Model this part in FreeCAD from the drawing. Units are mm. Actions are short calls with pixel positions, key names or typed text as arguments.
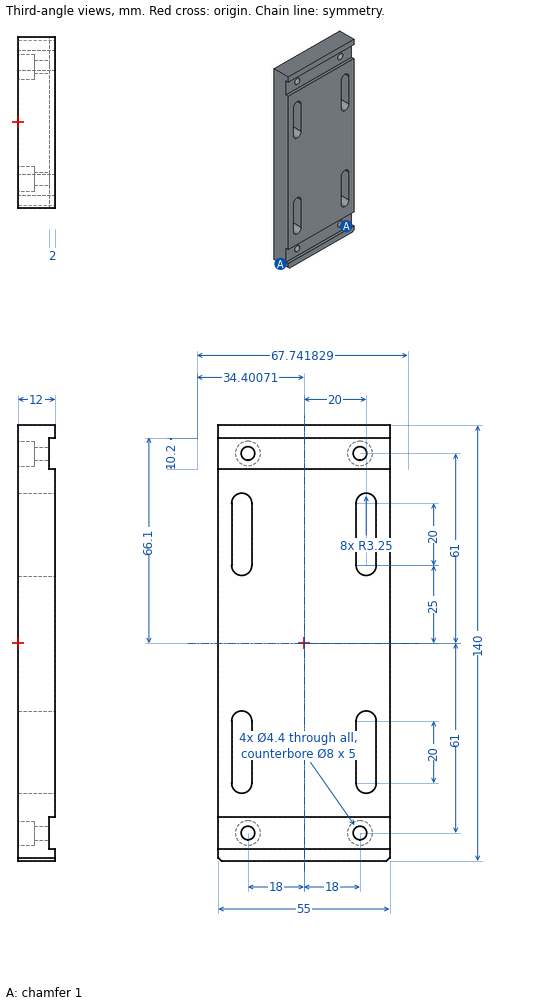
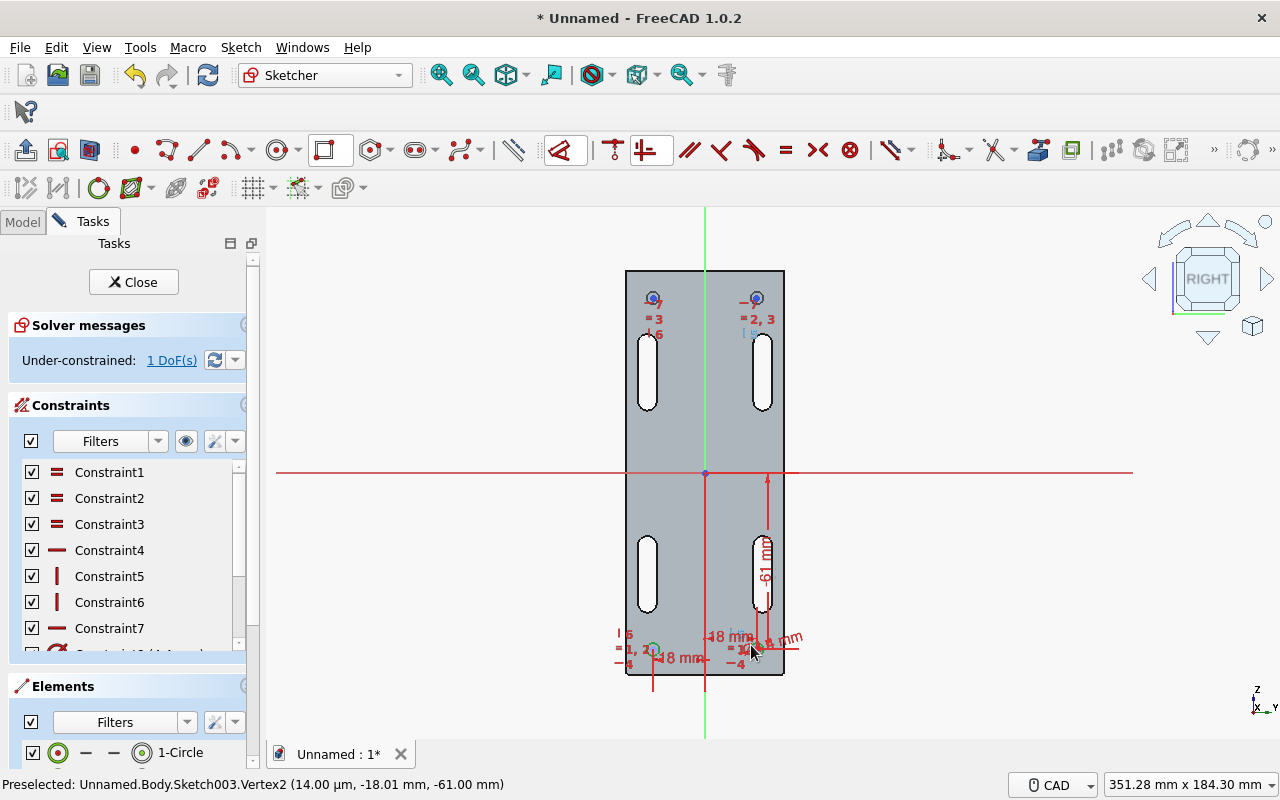
click(757, 298)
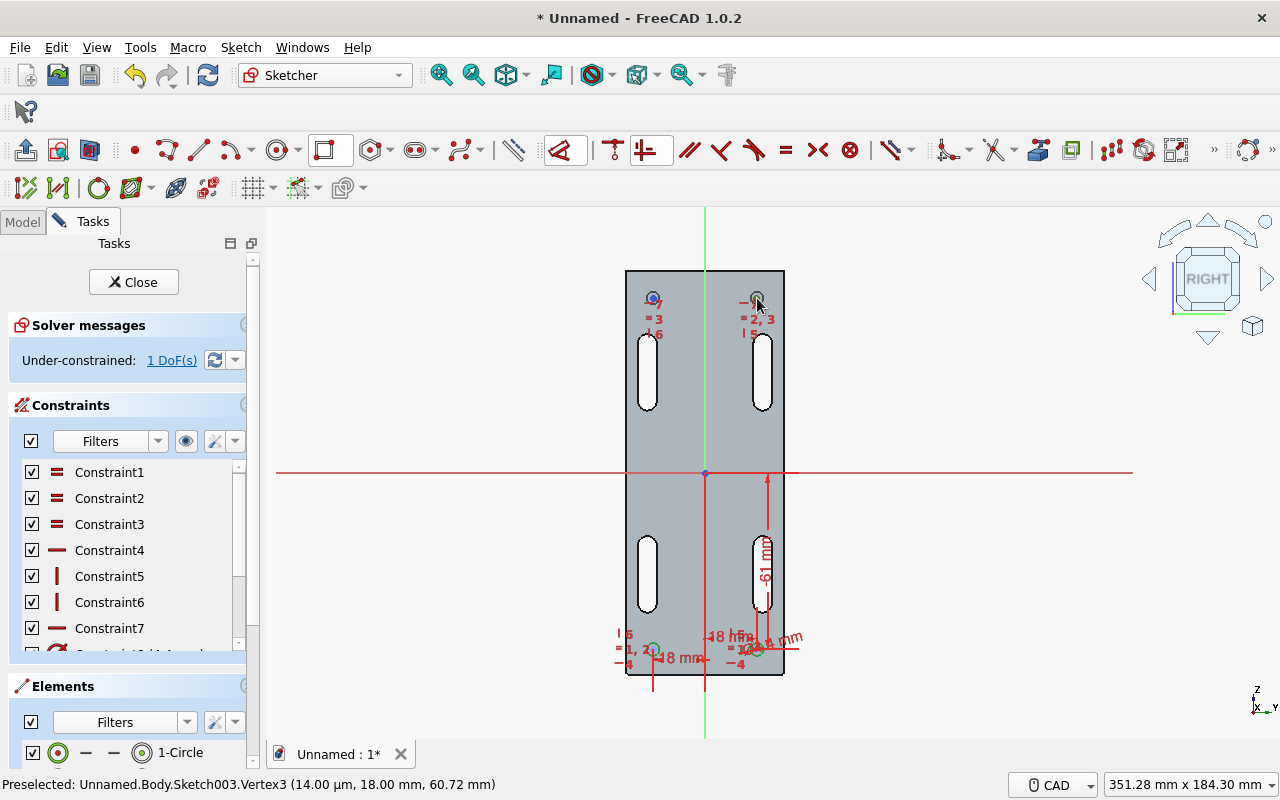
click(582, 150)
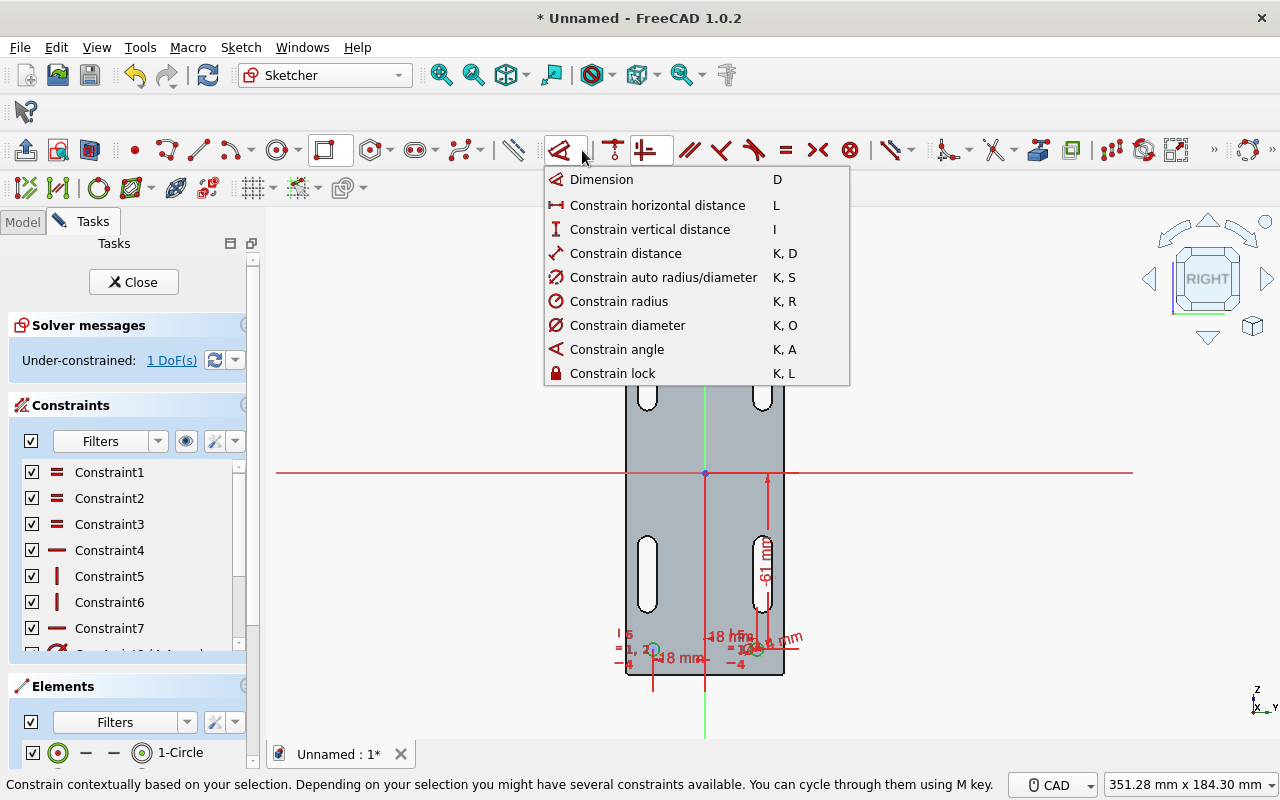
click(697, 229)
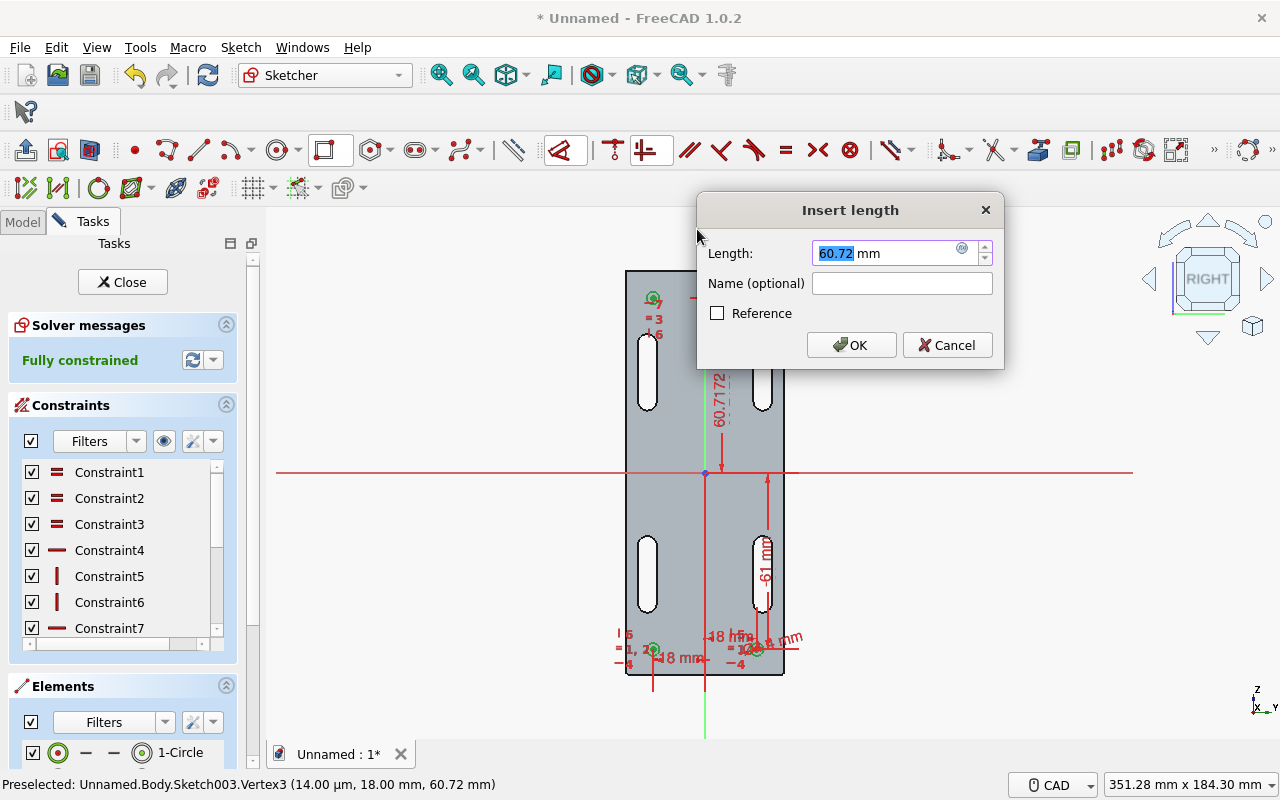
text(61)
key(Return)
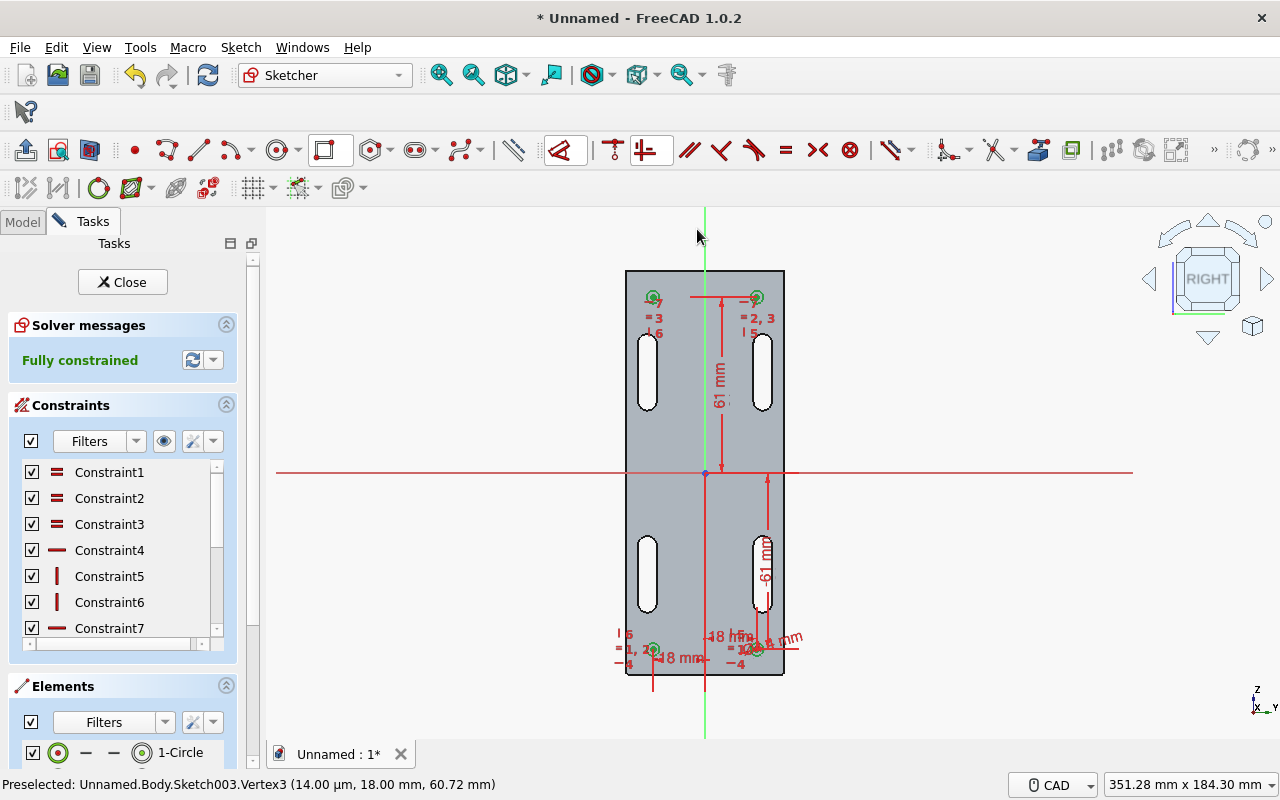
click(123, 282)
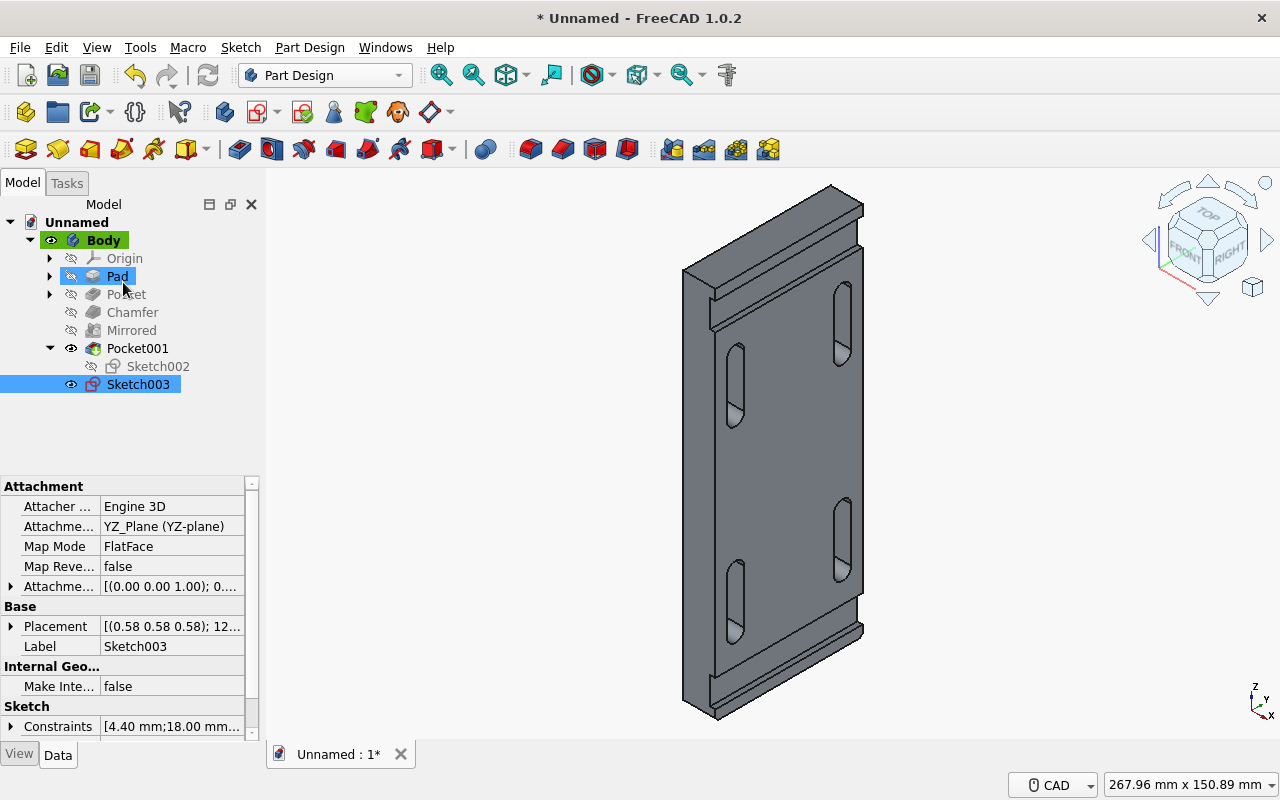
click(272, 150)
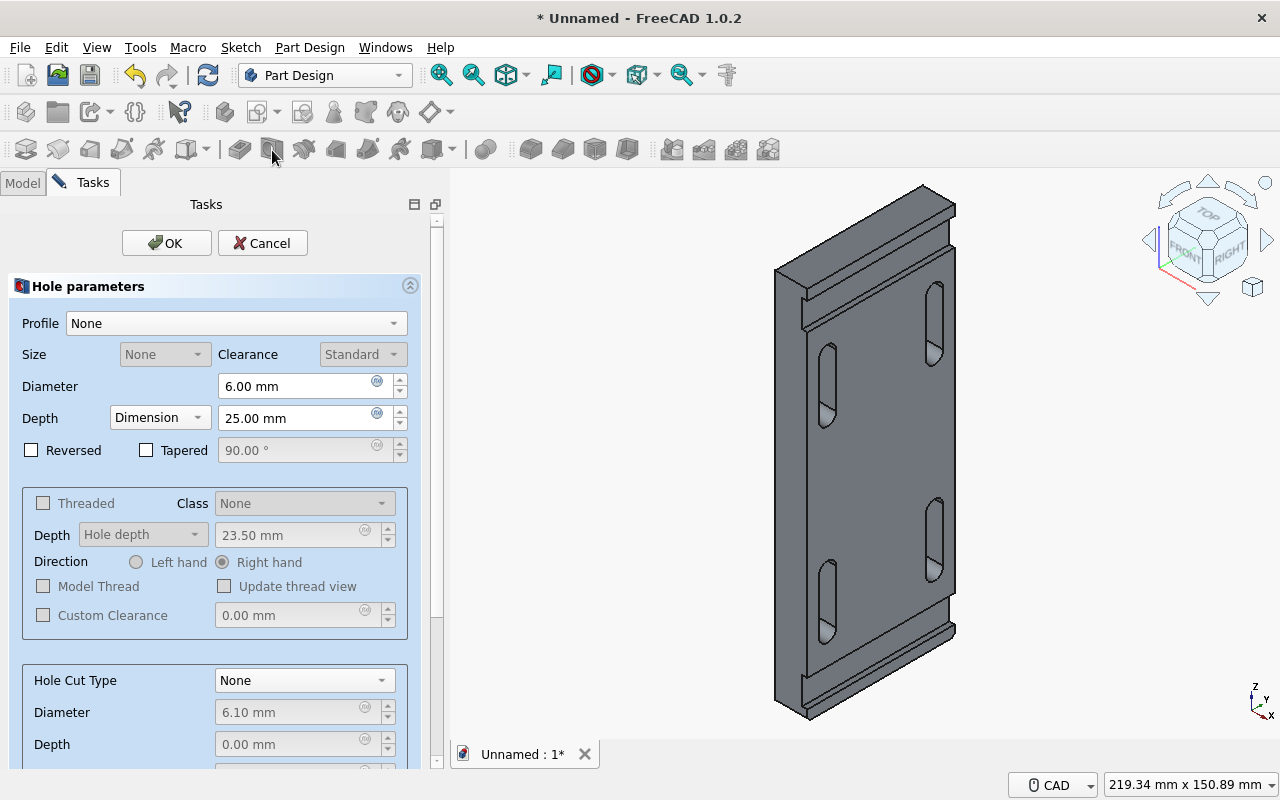
triple_click(305, 386)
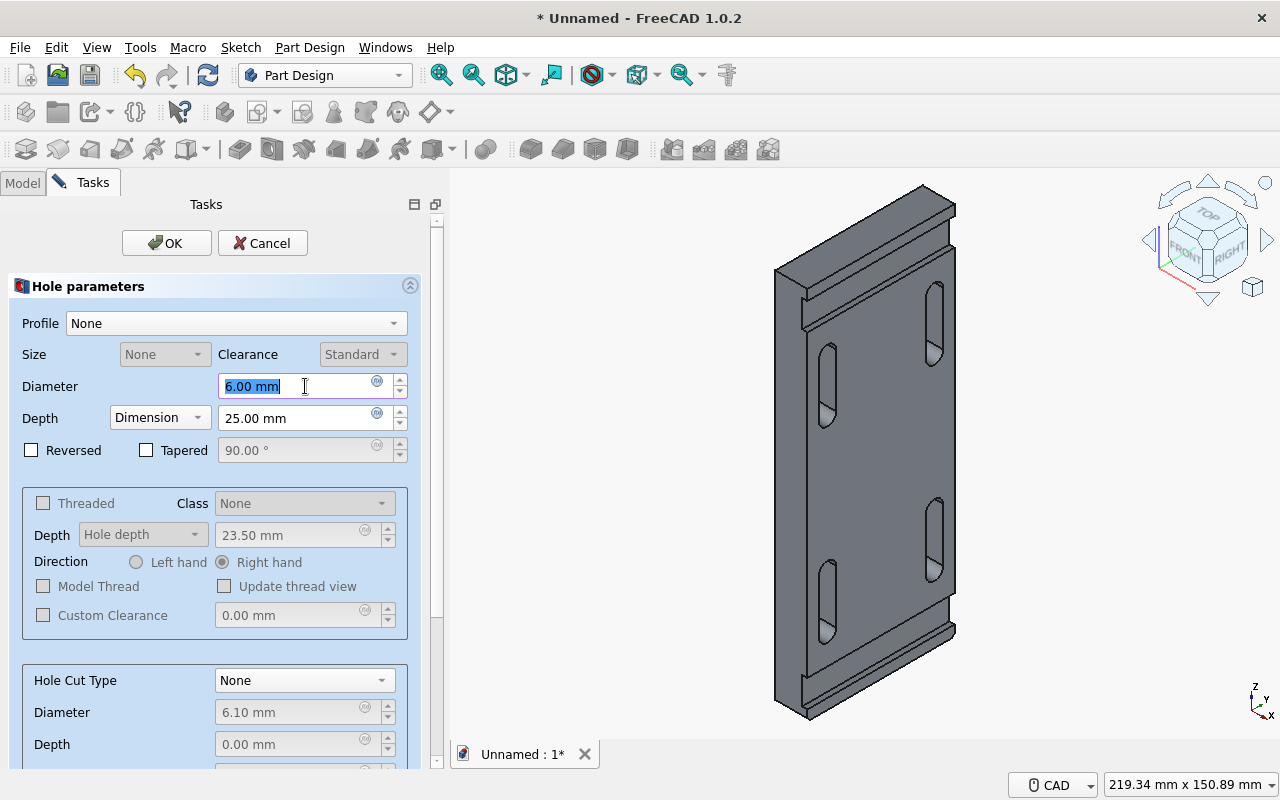
text(4.4)
key(Tab)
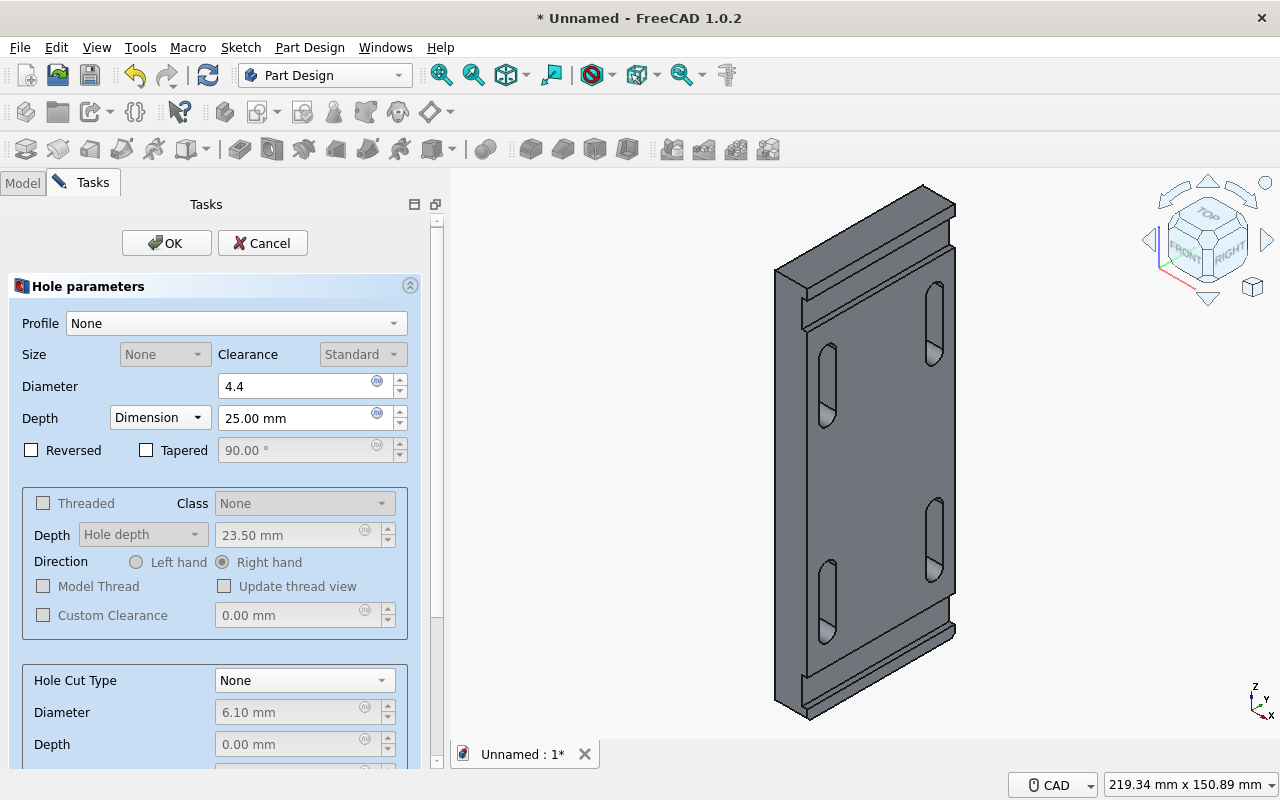
click(161, 418)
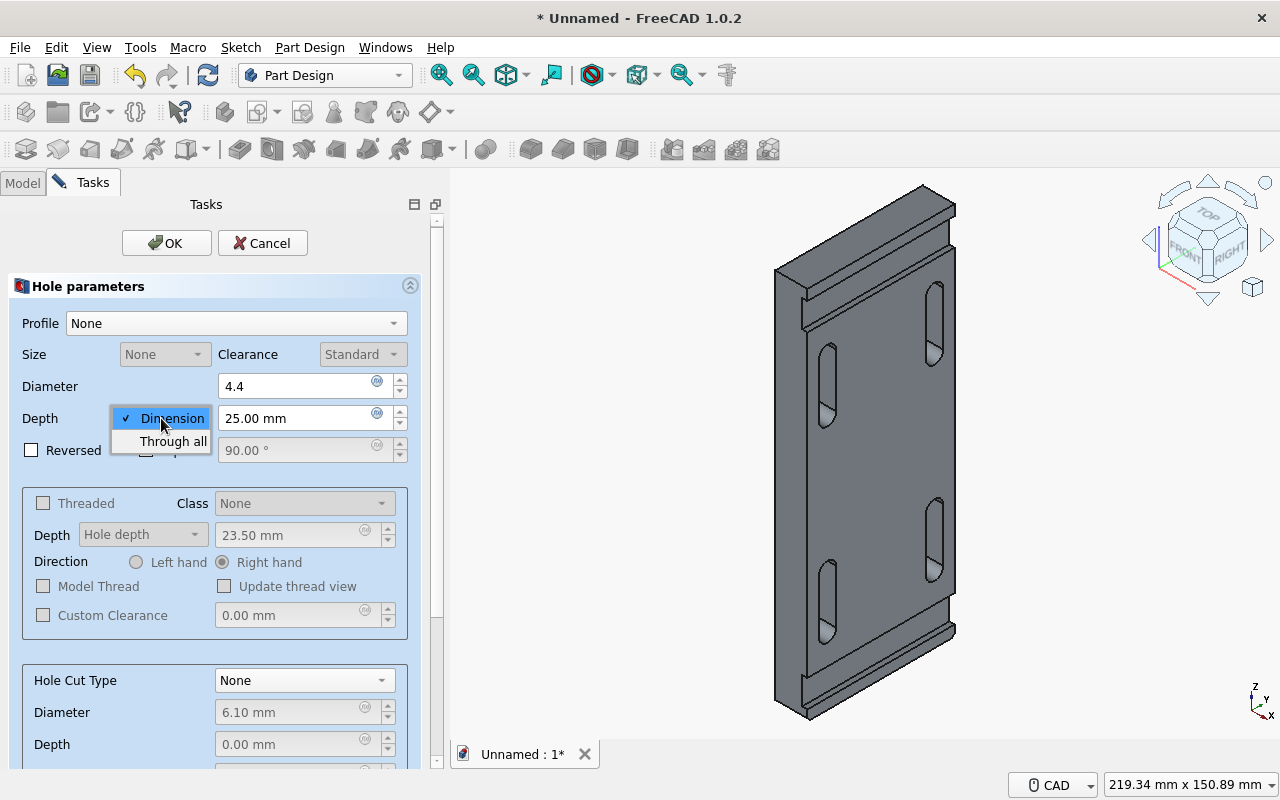
click(160, 442)